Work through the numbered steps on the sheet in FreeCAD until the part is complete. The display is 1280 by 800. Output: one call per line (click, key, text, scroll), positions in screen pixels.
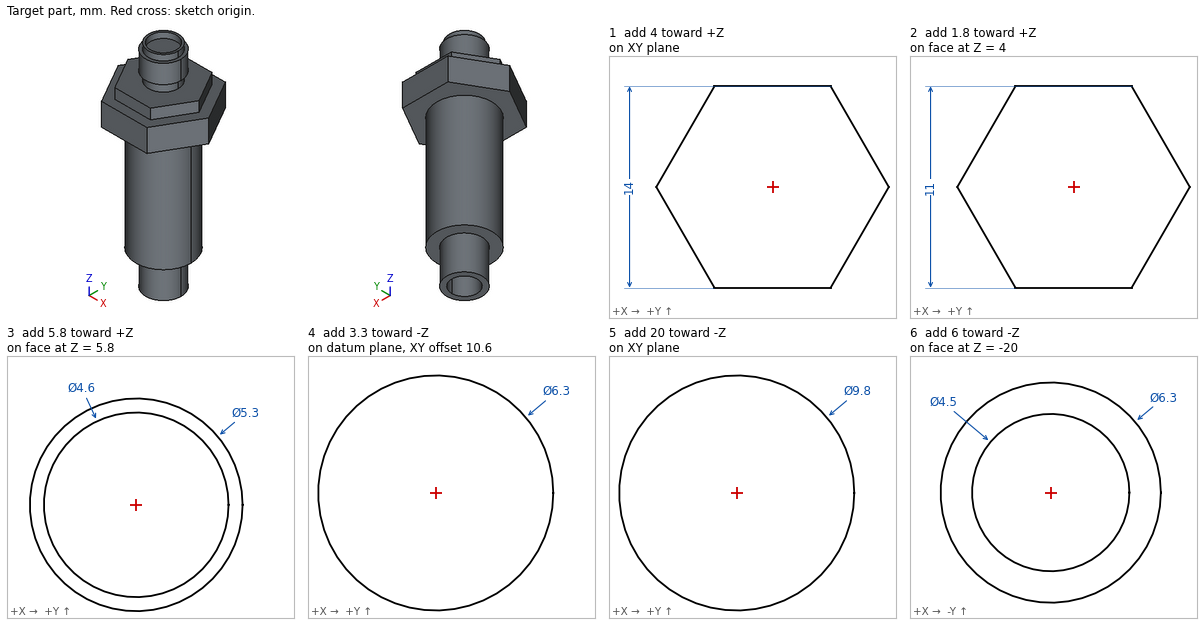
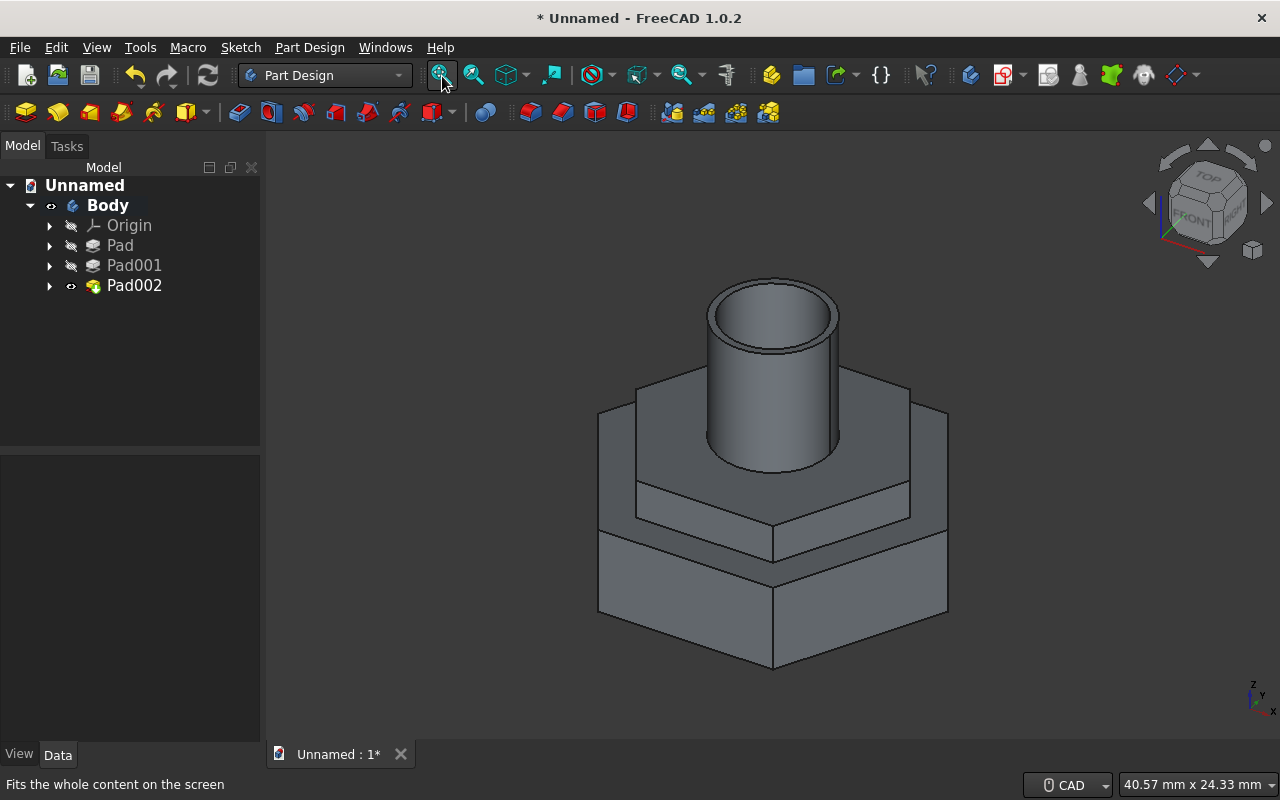
click(50, 226)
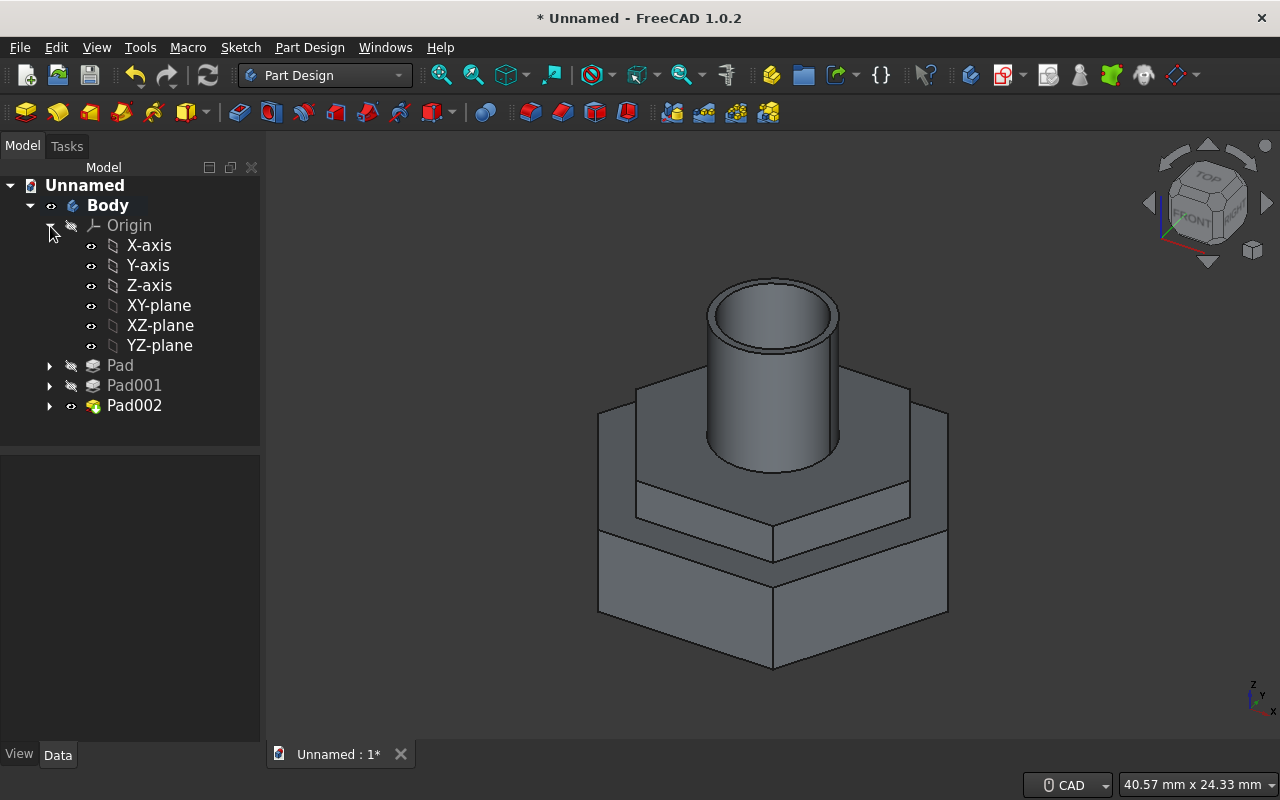
click(136, 306)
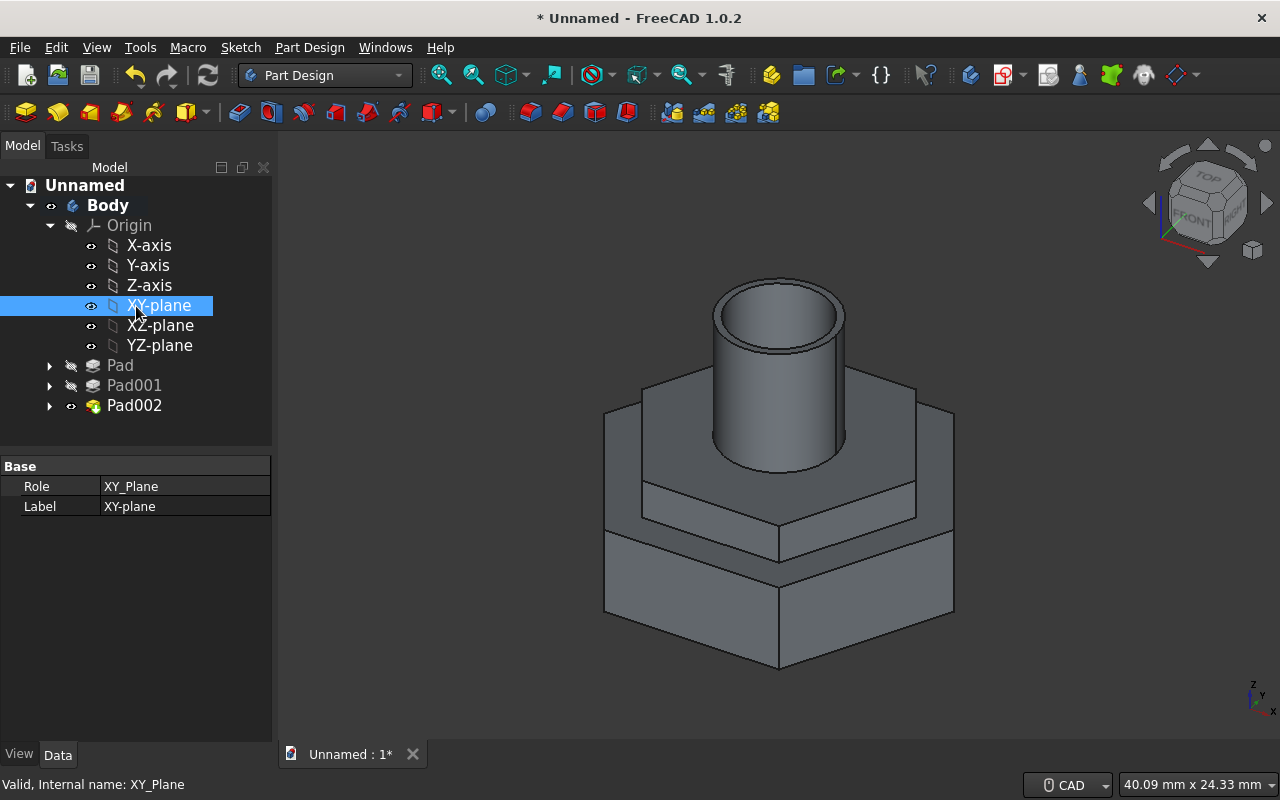
click(1176, 76)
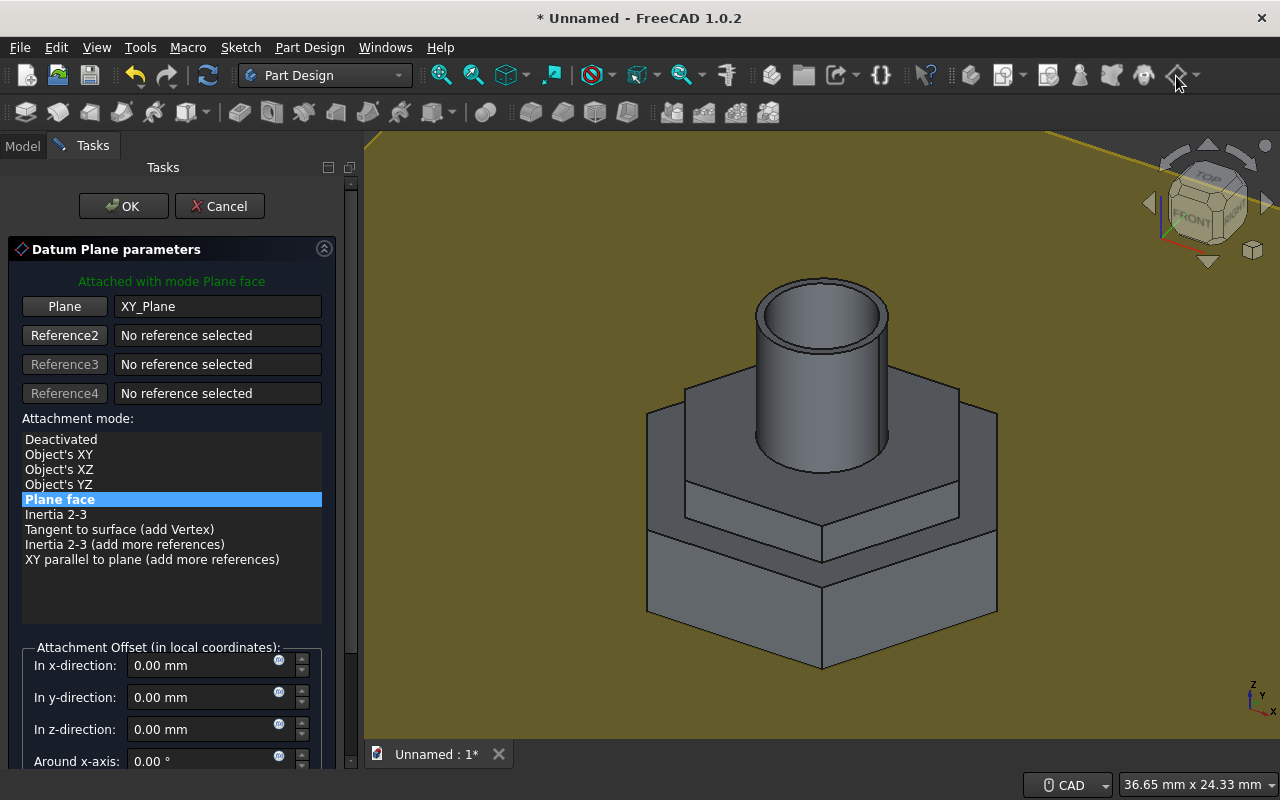
triple_click(210, 729)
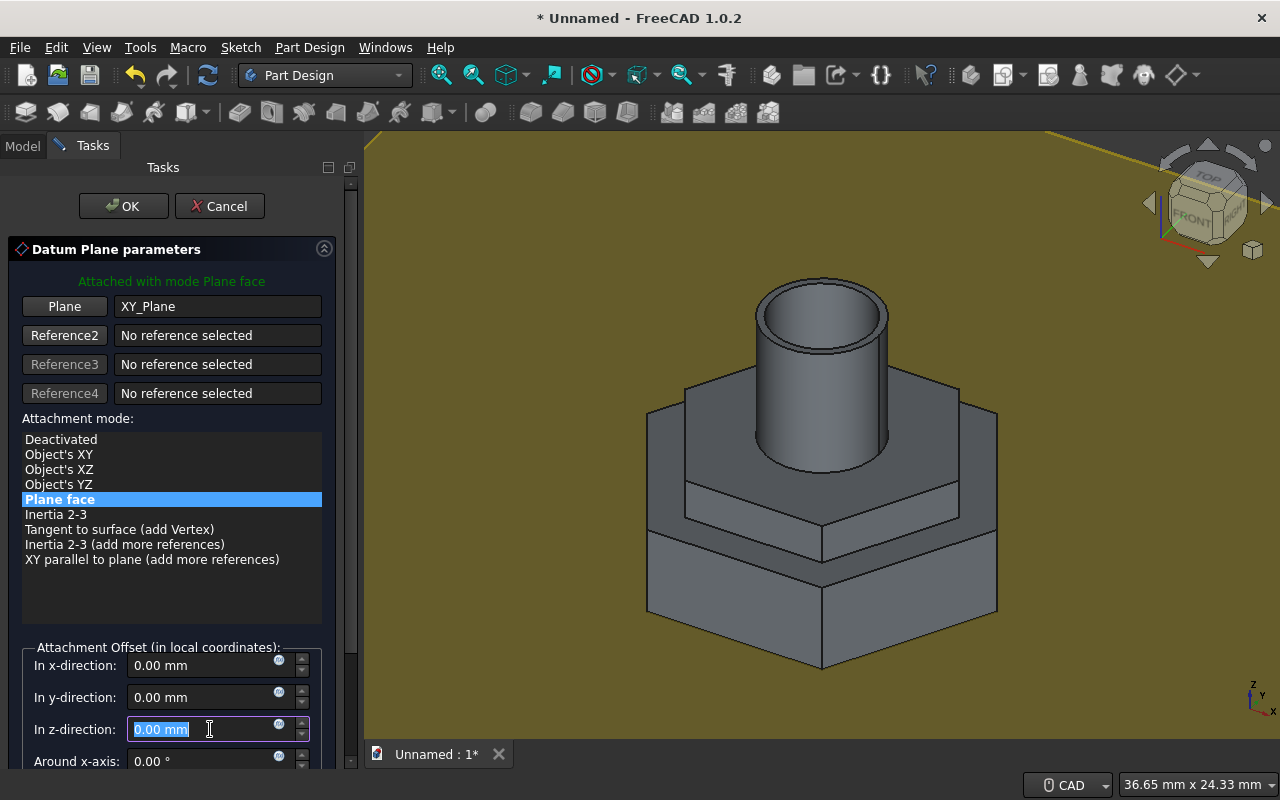
text(10.6)
key(Tab)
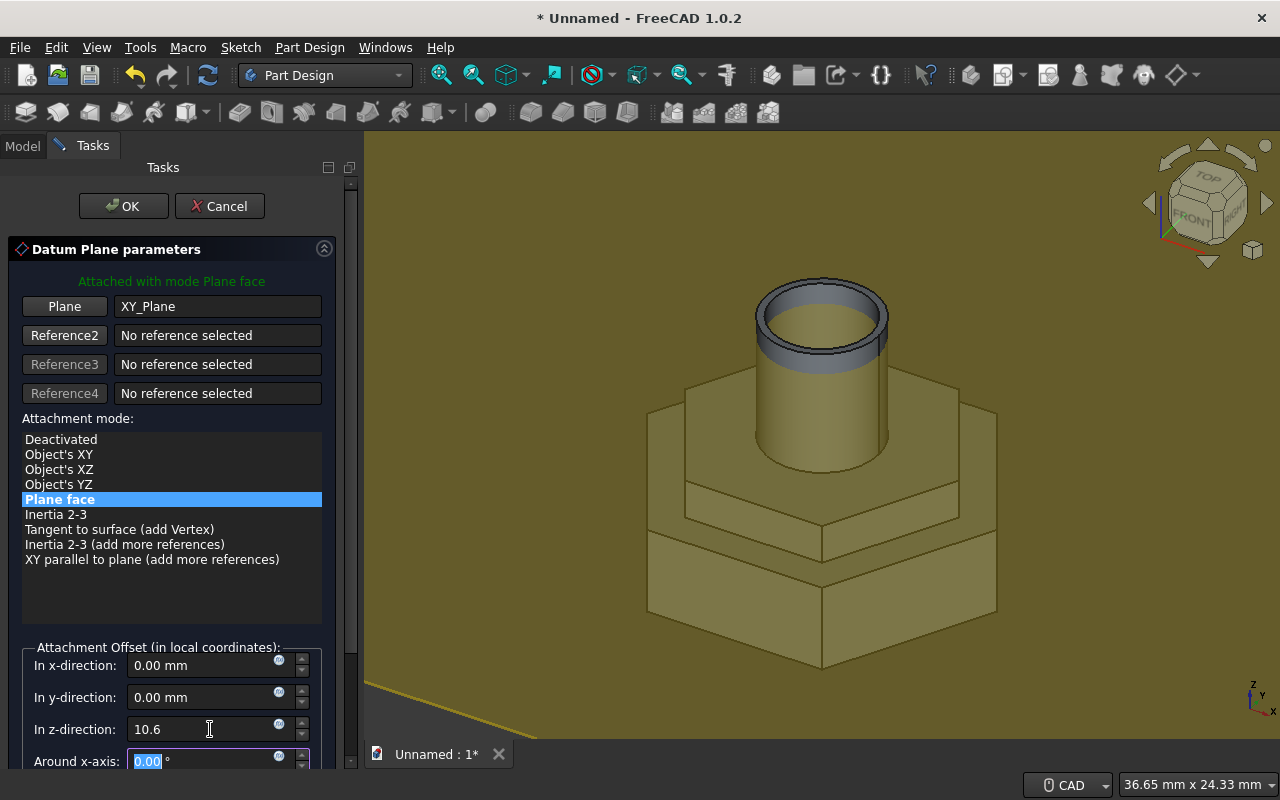
click(124, 206)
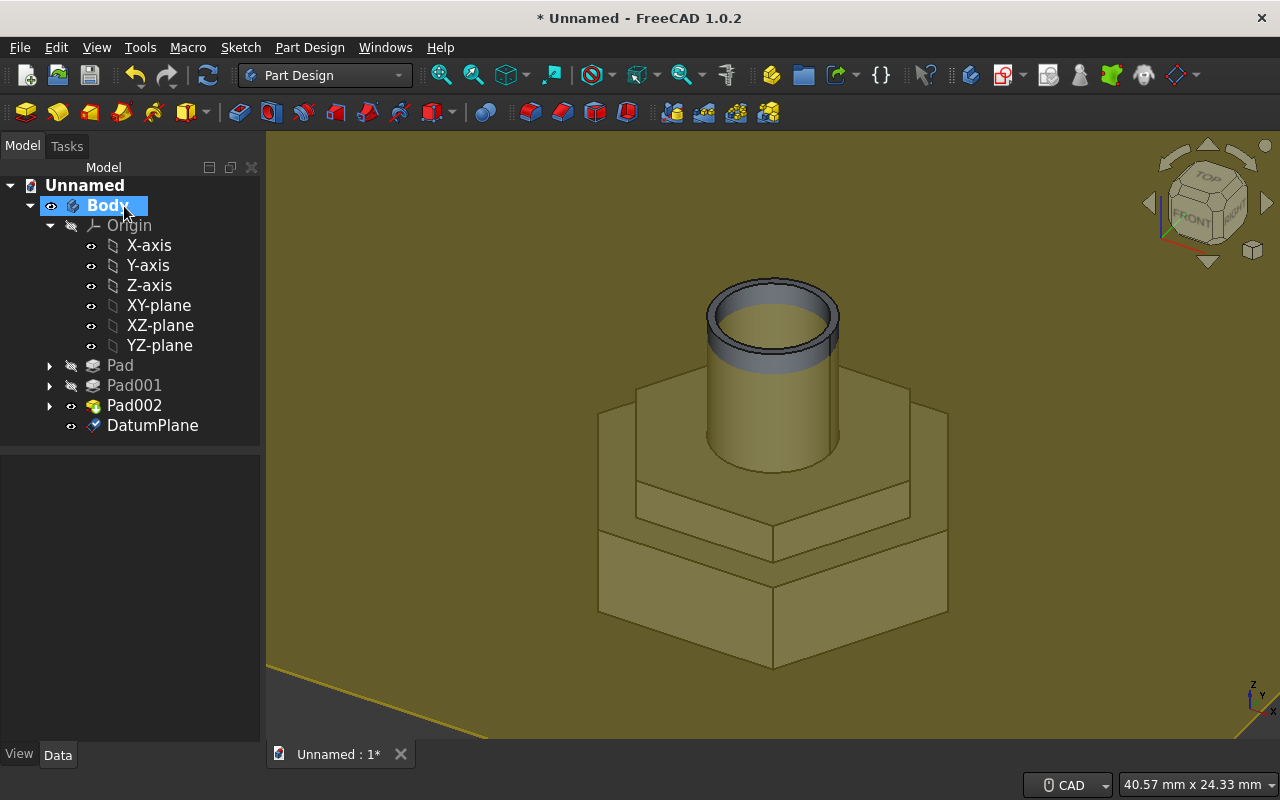
click(116, 426)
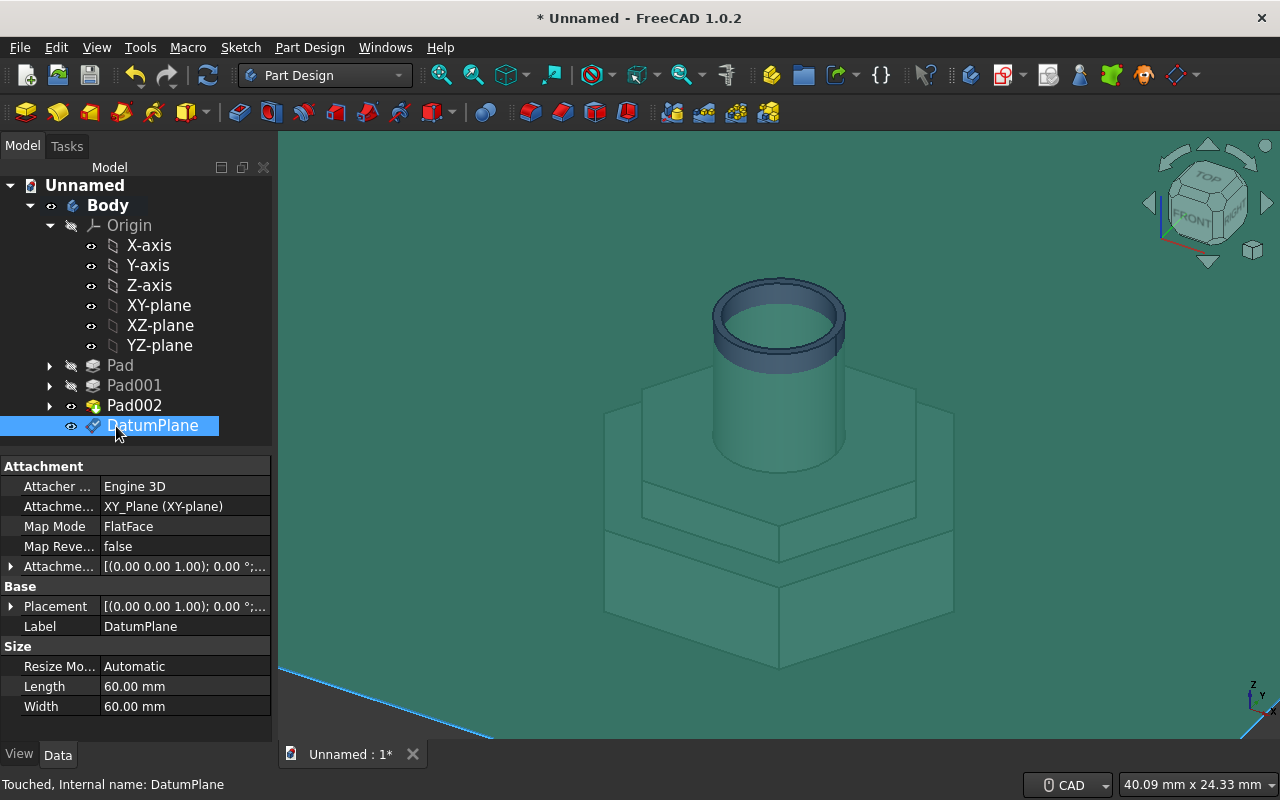
click(1004, 76)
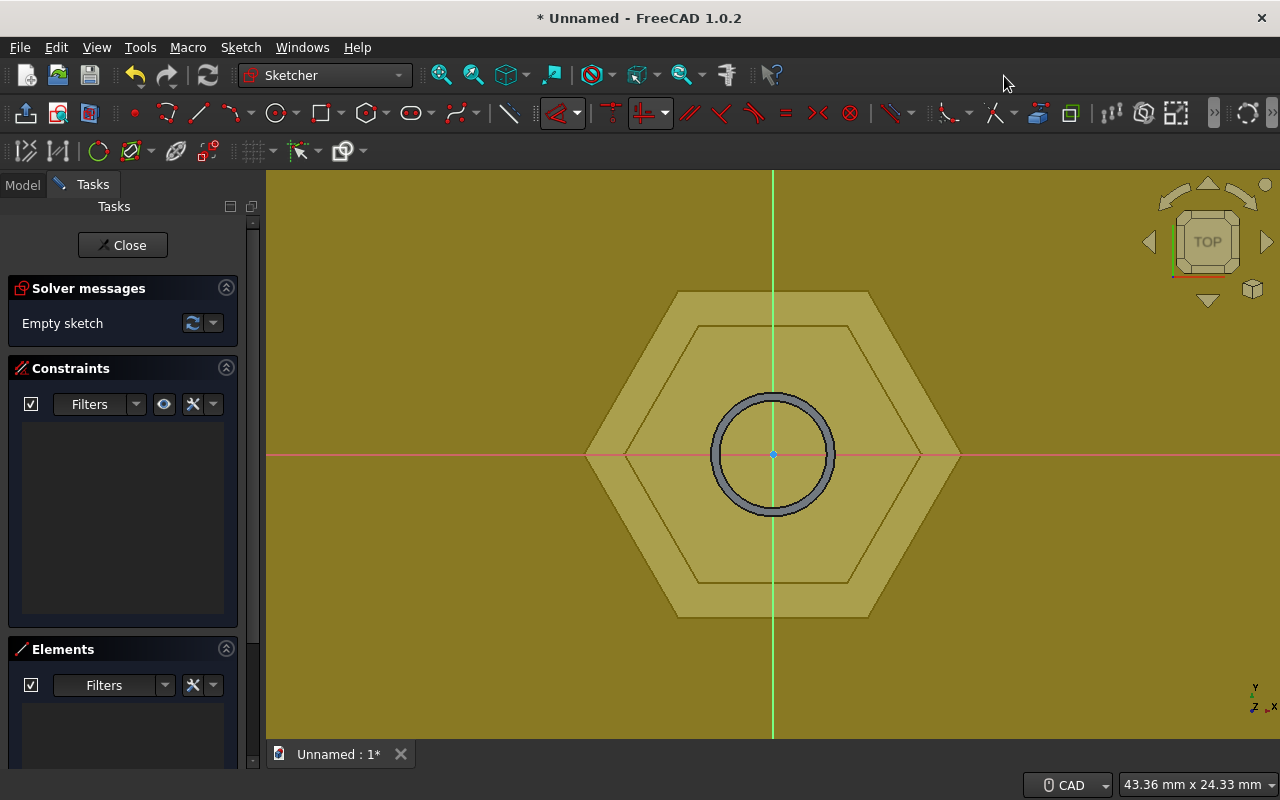
click(90, 114)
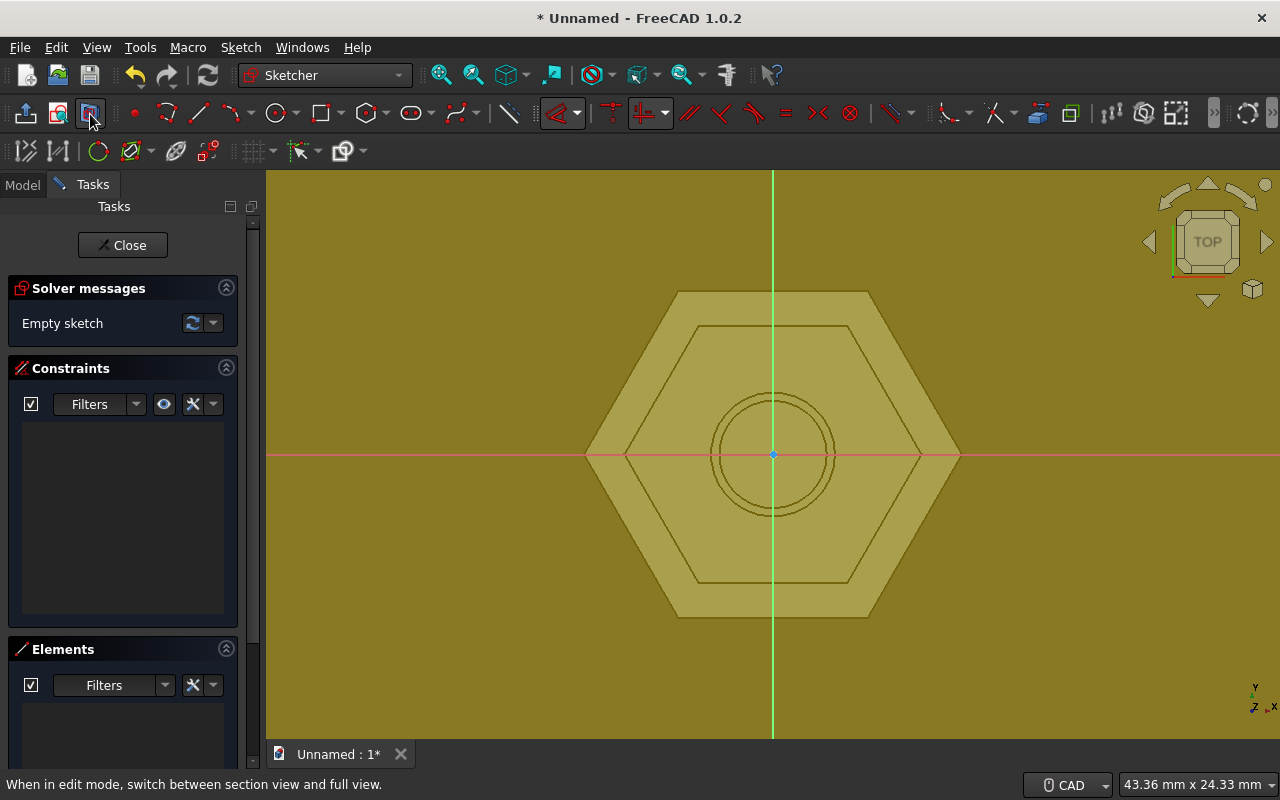
scroll(829, 455, up, 4)